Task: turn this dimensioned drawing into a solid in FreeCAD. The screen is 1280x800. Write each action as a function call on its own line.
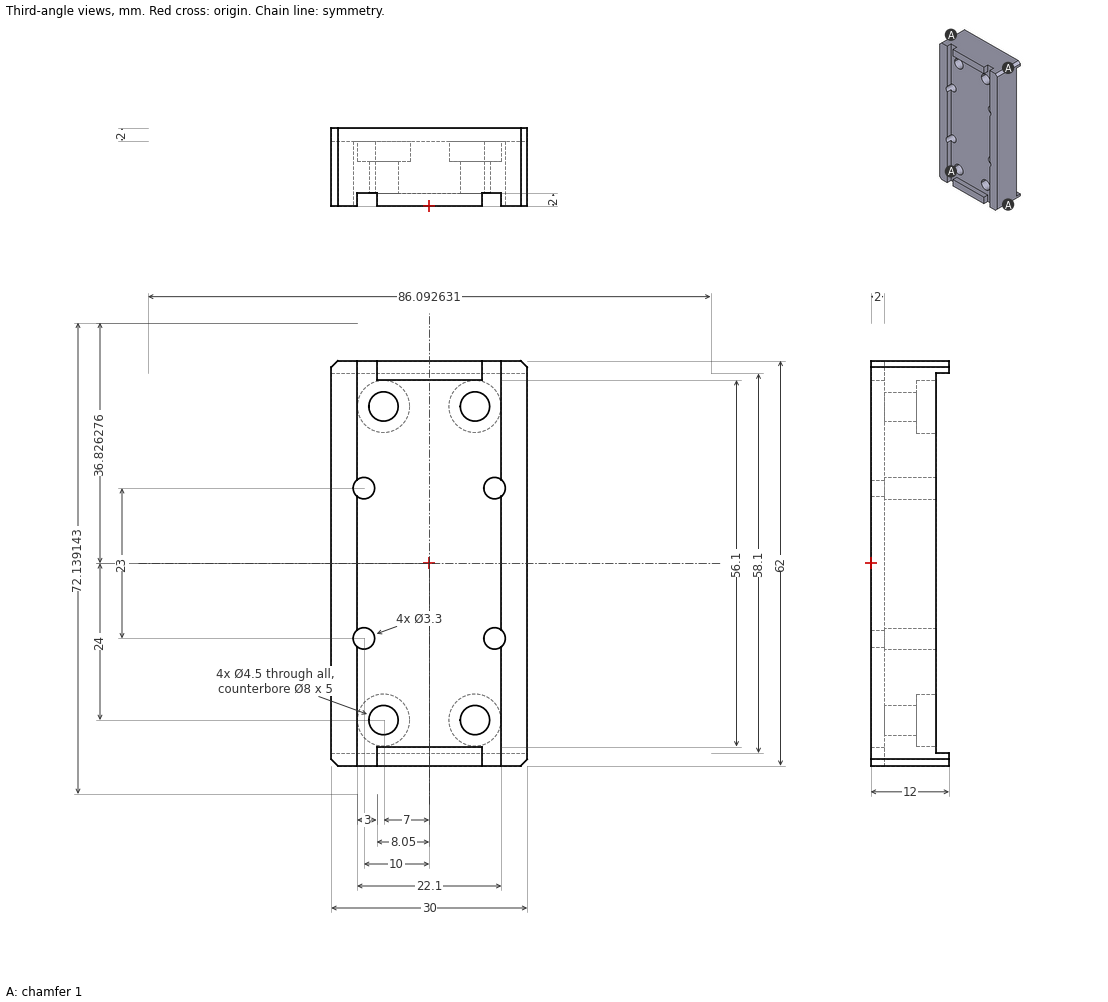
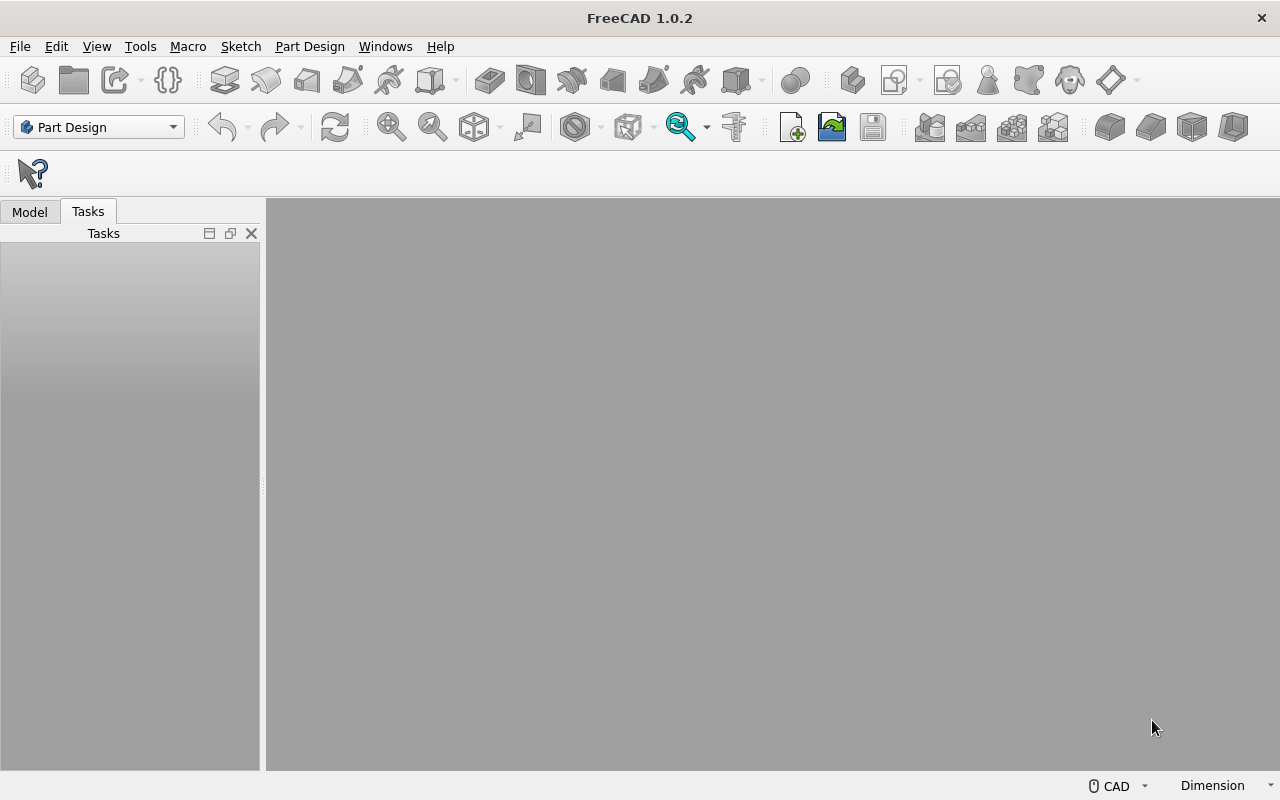
click(791, 128)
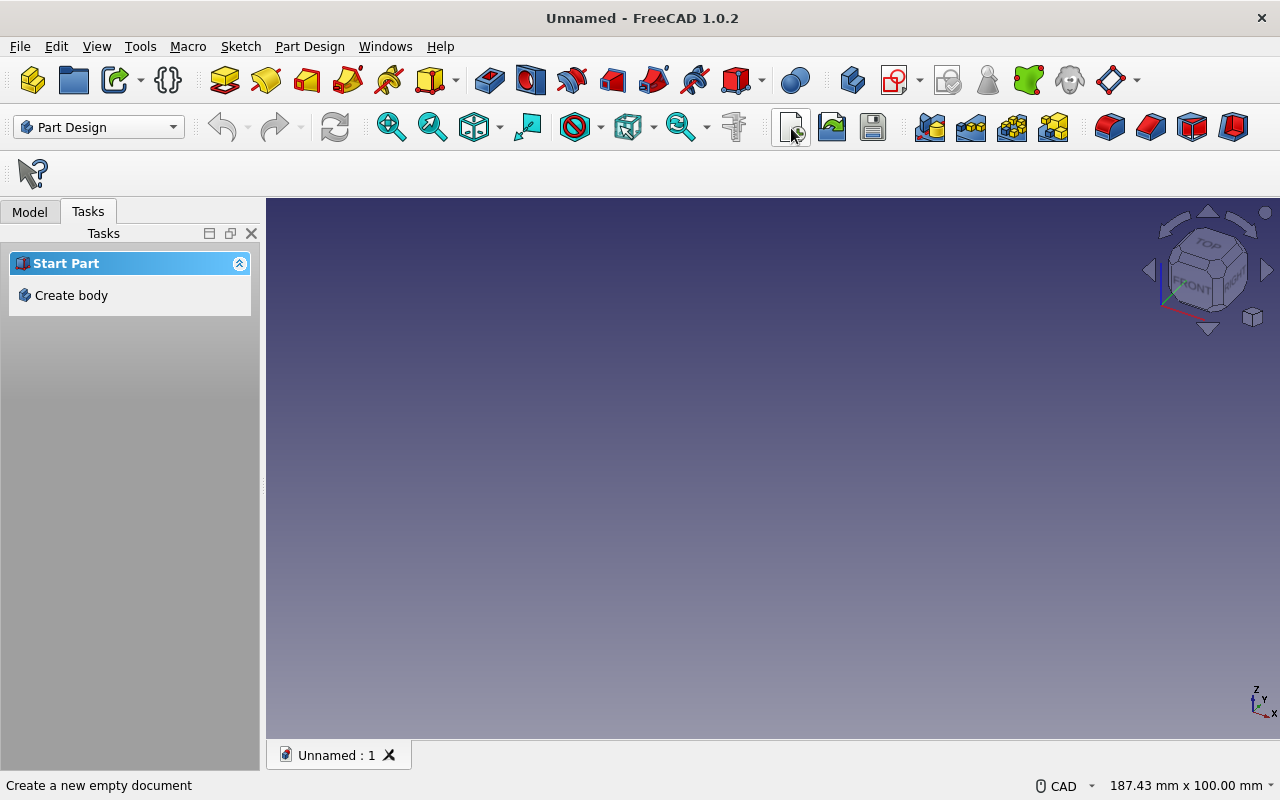
click(894, 80)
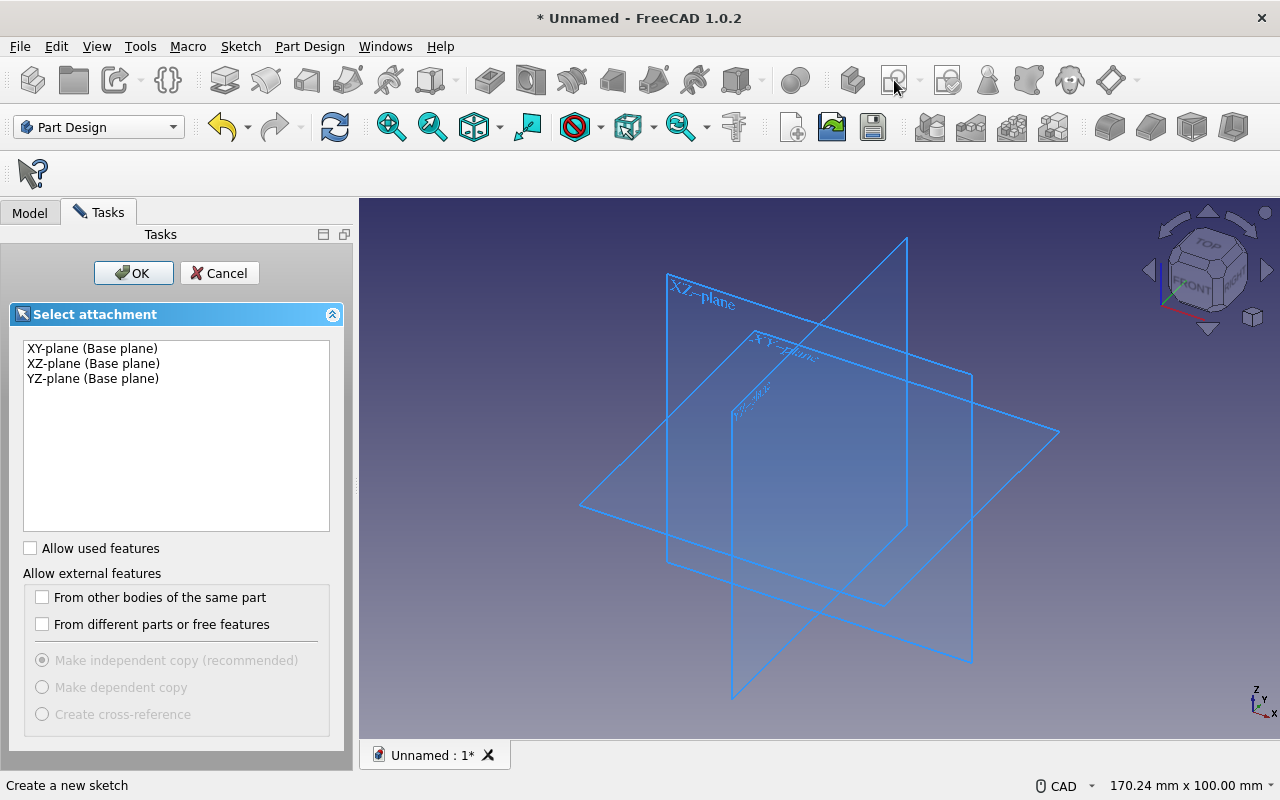
click(84, 364)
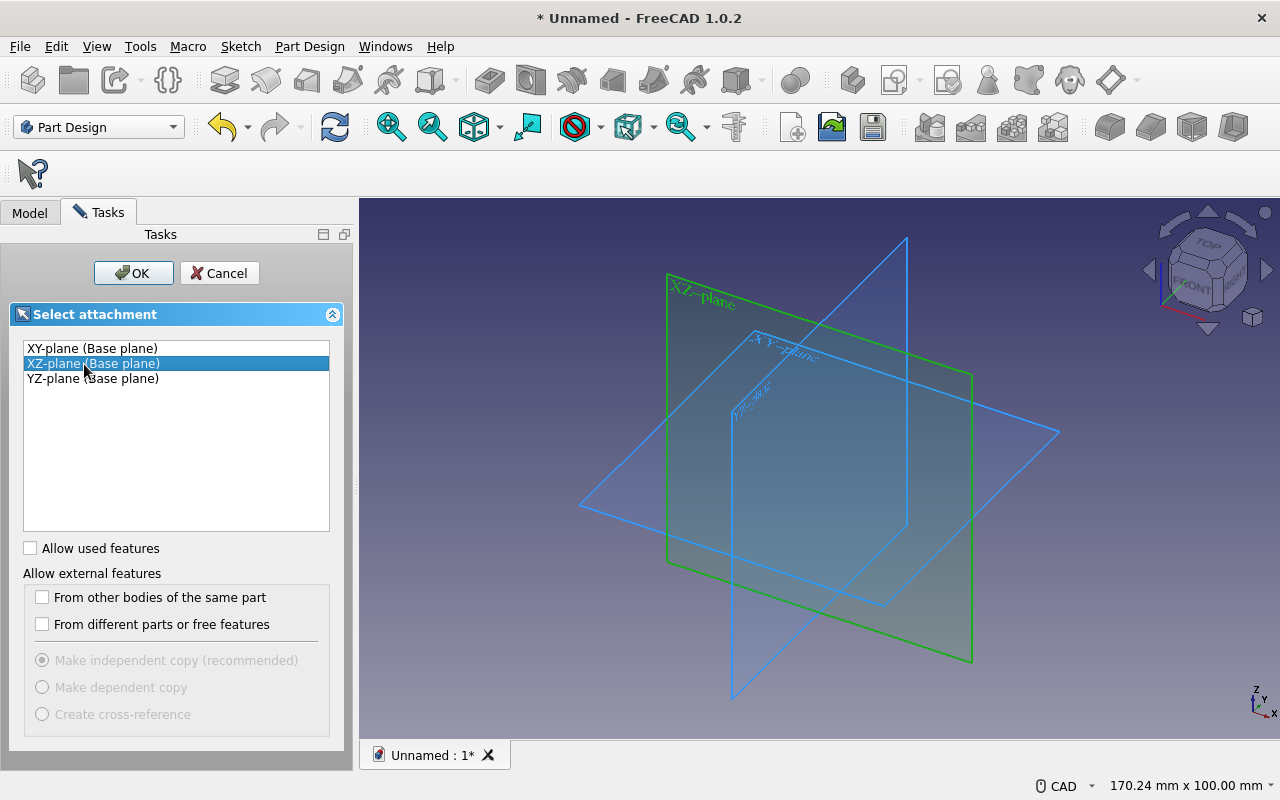
click(134, 273)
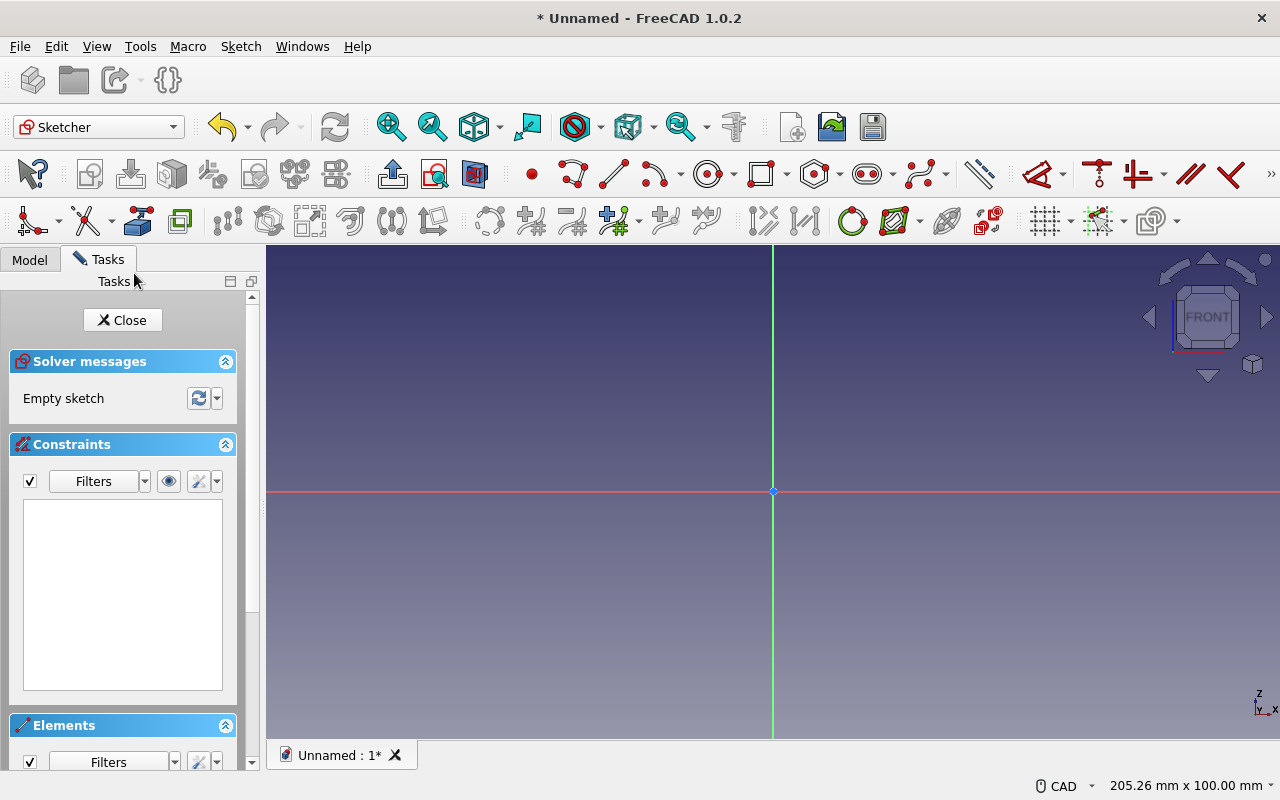
key(g)
key(v)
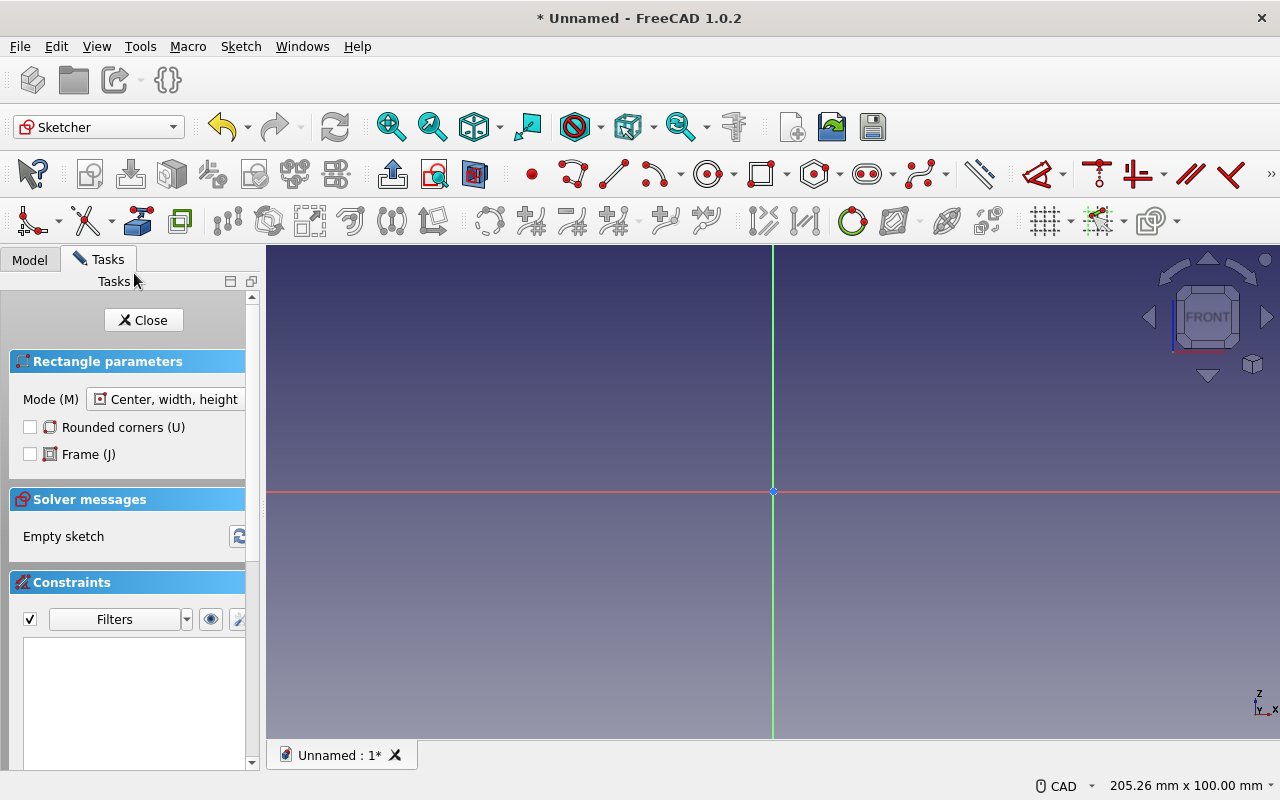
click(773, 492)
click(847, 339)
key(Escape)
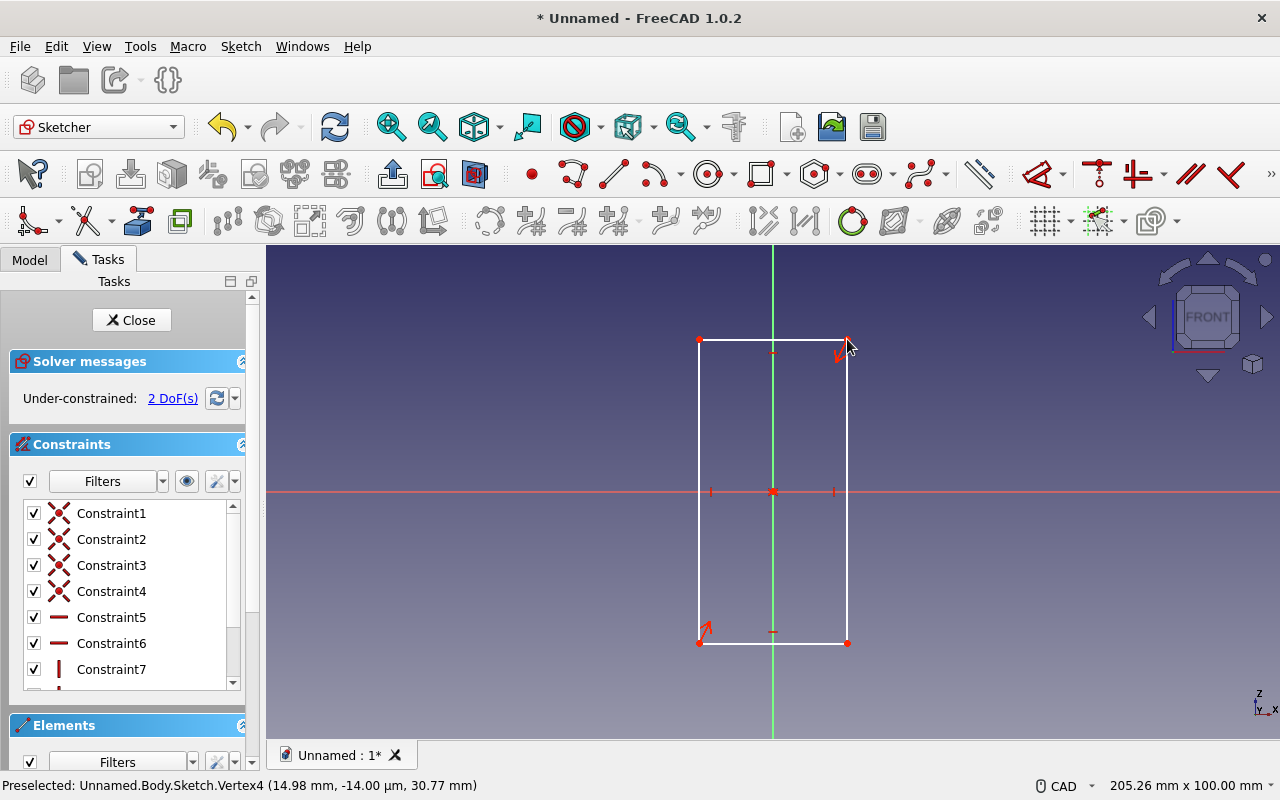
click(743, 644)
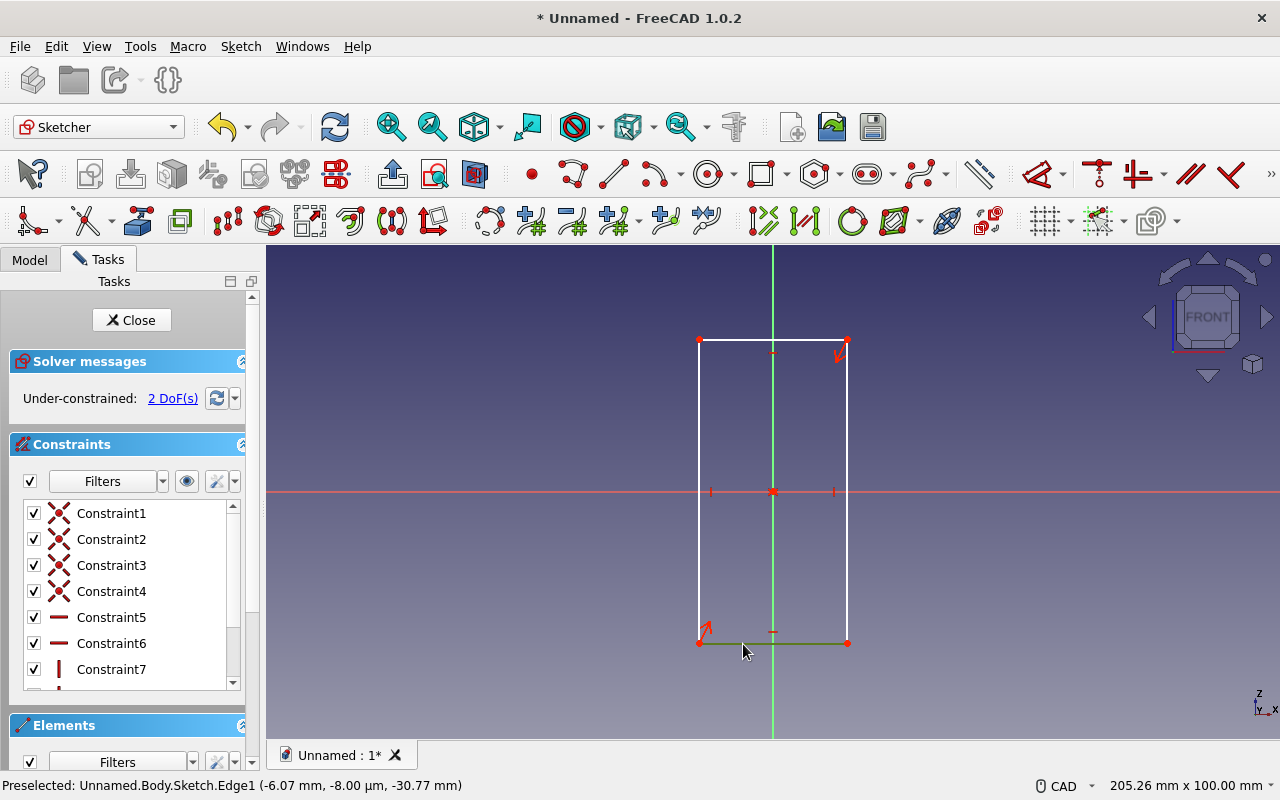
click(1062, 174)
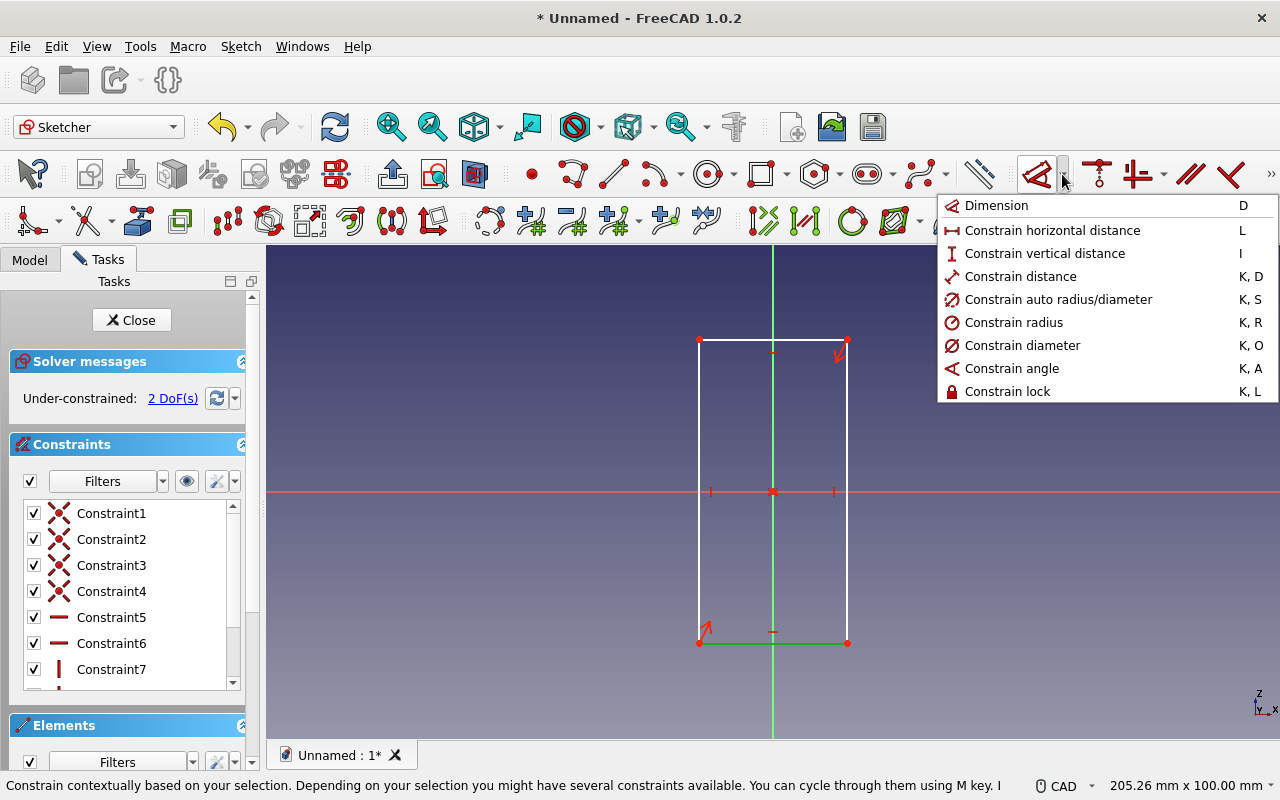
click(1108, 230)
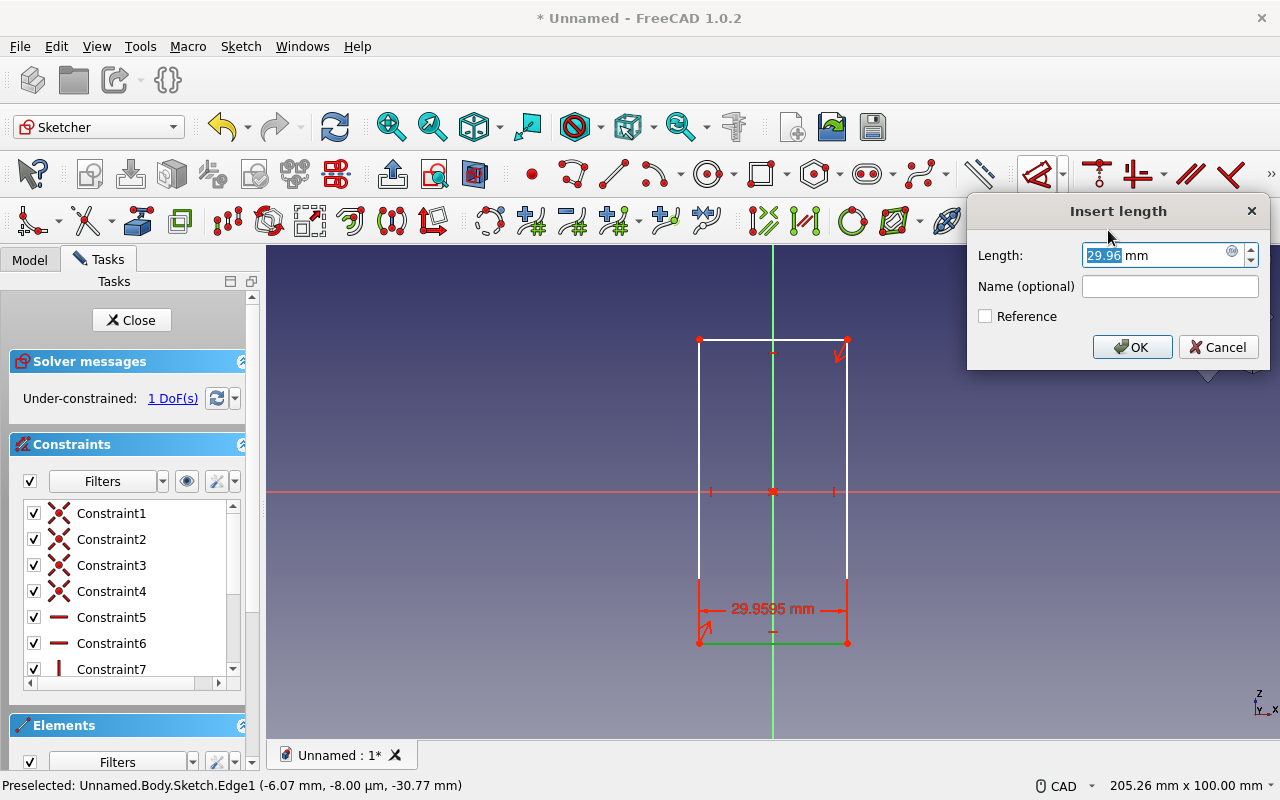
text(30)
key(Return)